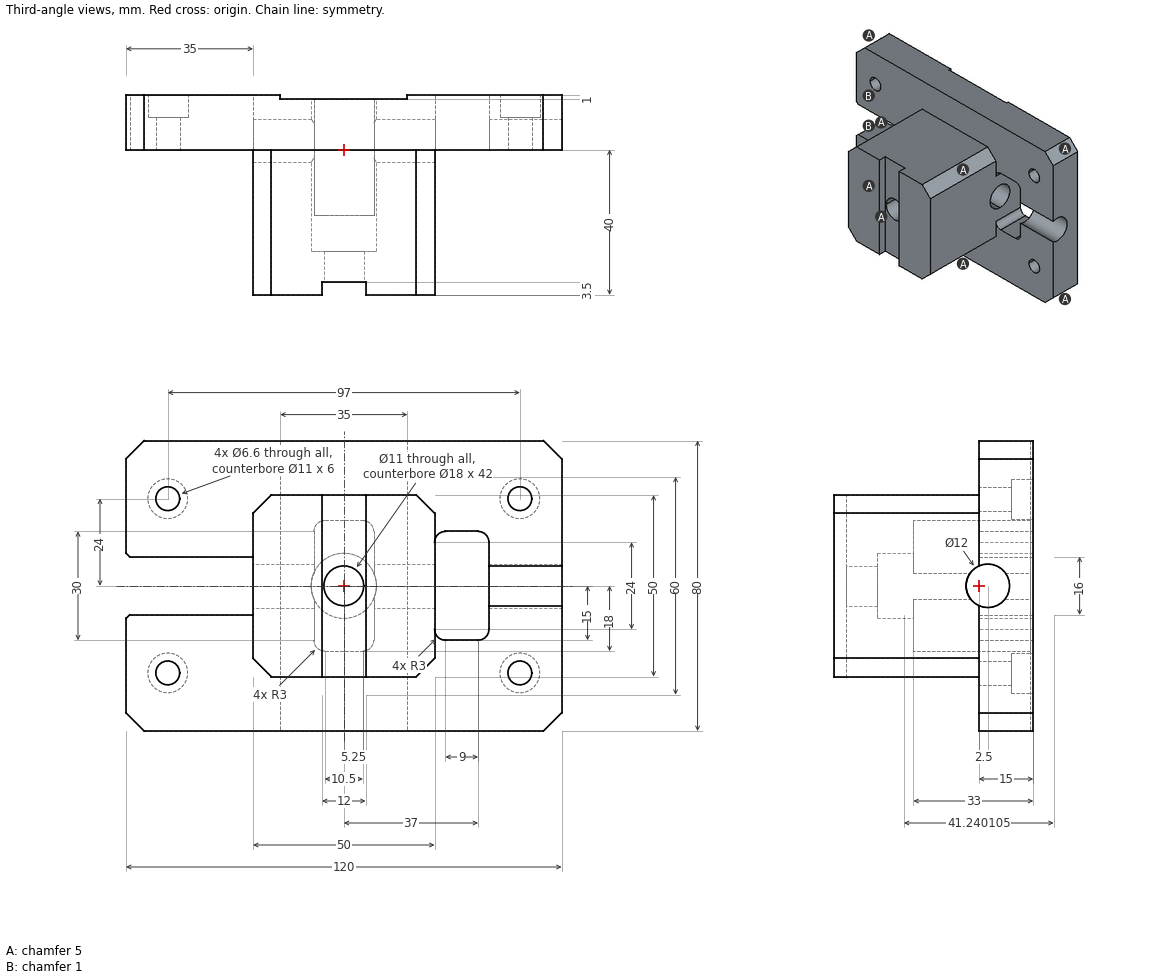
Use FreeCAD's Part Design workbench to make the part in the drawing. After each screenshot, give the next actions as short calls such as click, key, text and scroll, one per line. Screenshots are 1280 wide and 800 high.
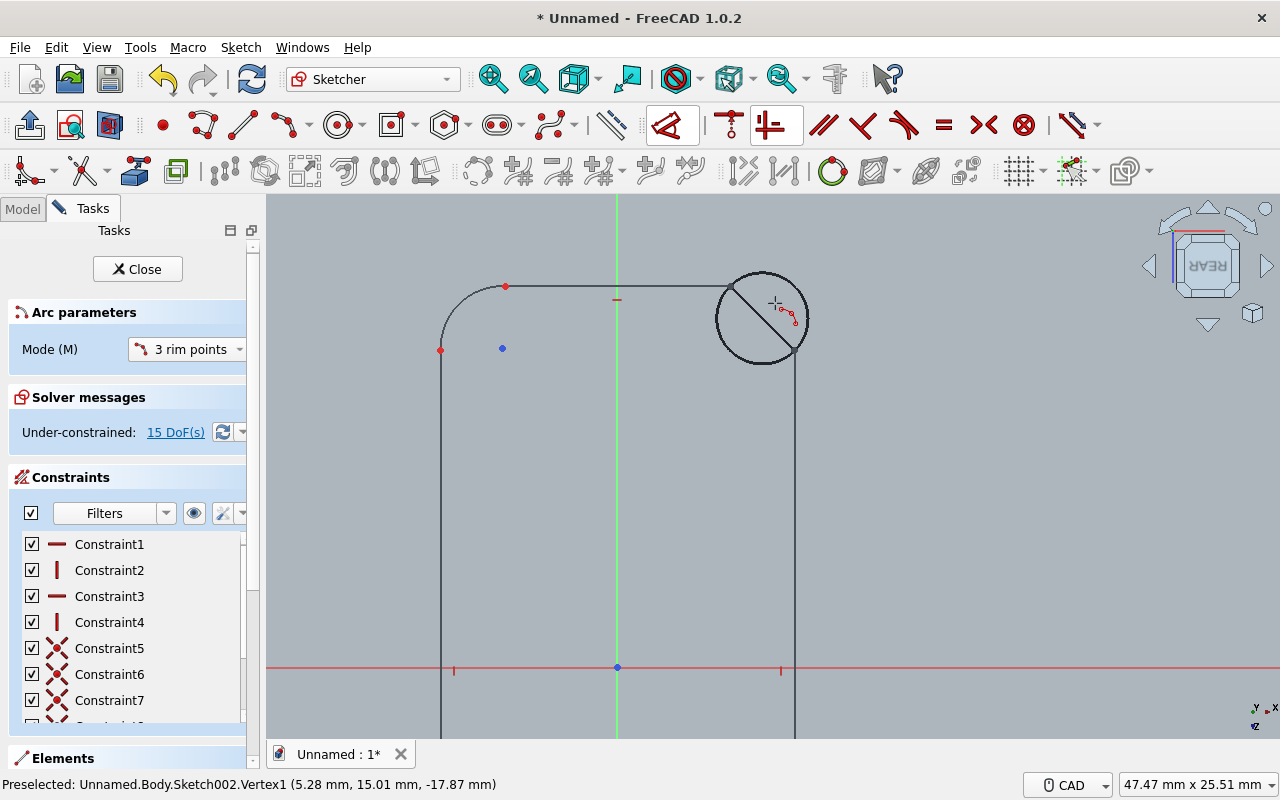
click(775, 302)
key(Escape)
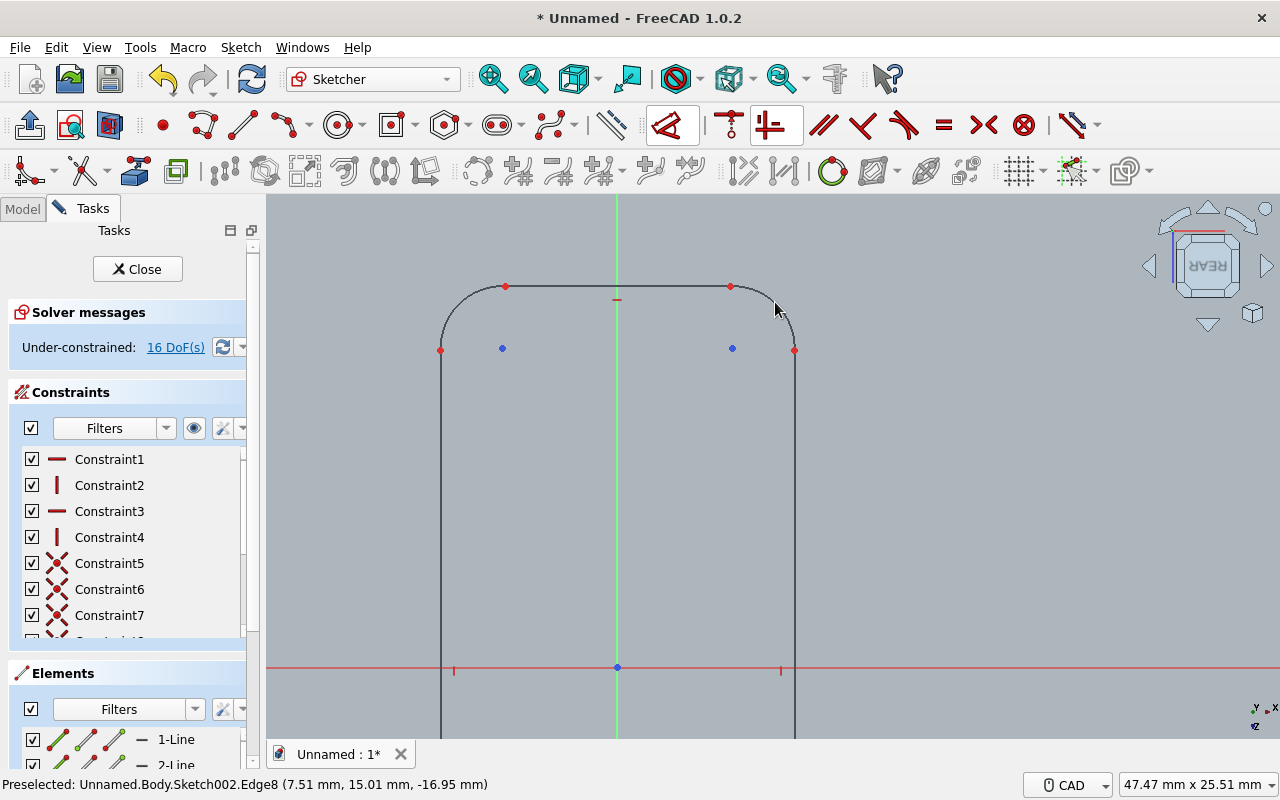
click(663, 286)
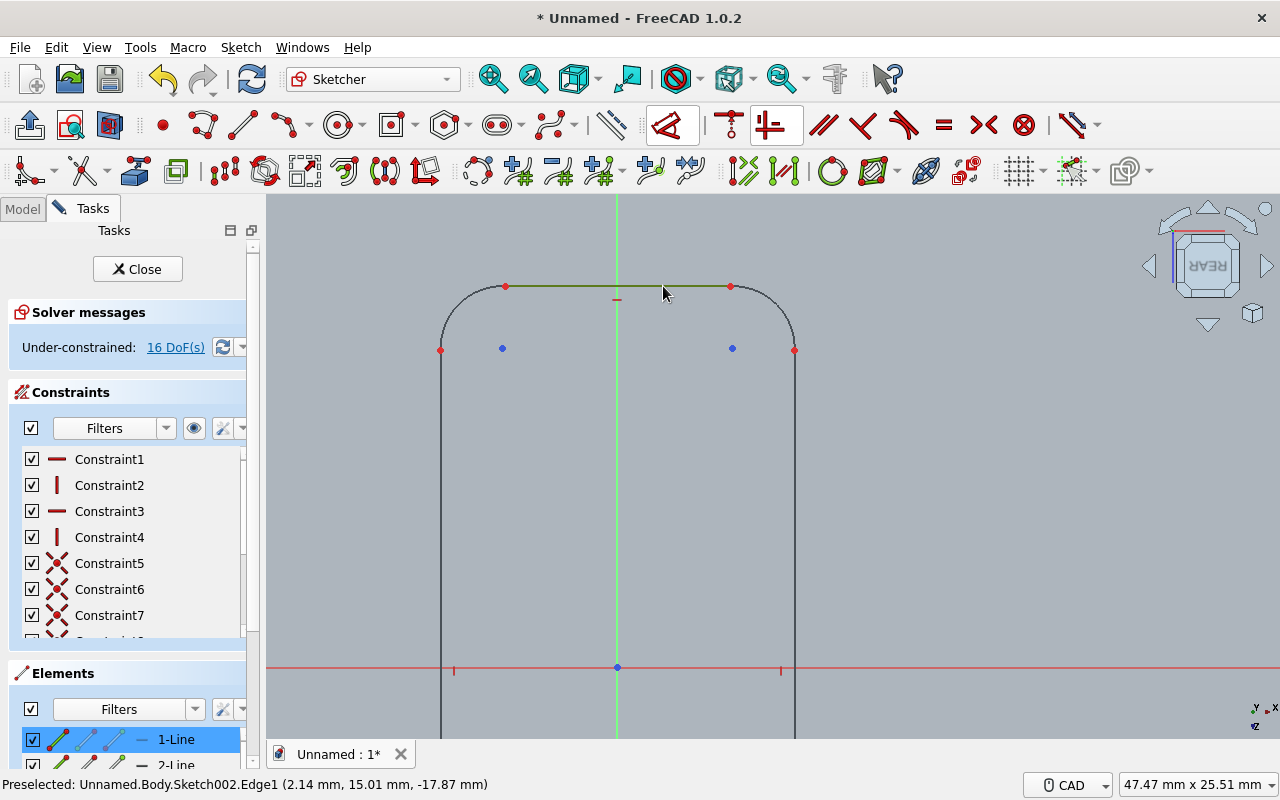
click(476, 292)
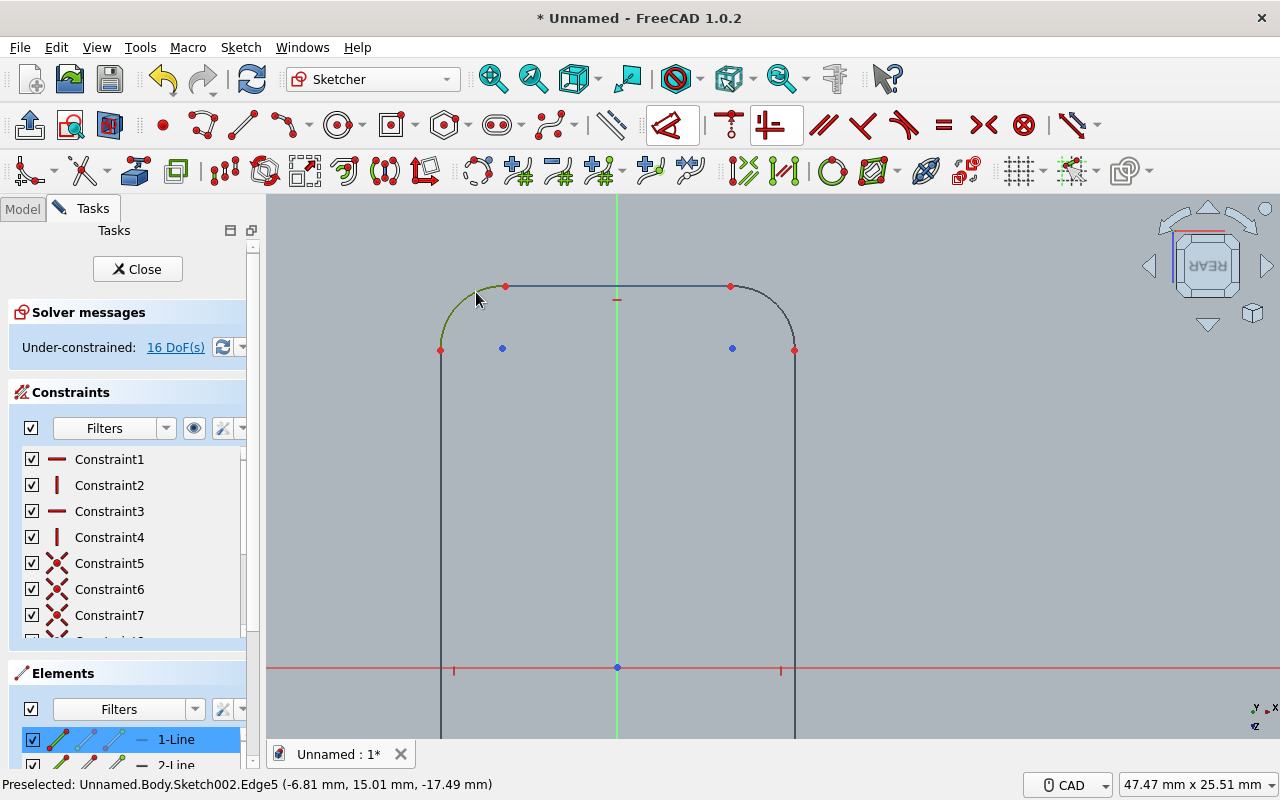
click(904, 126)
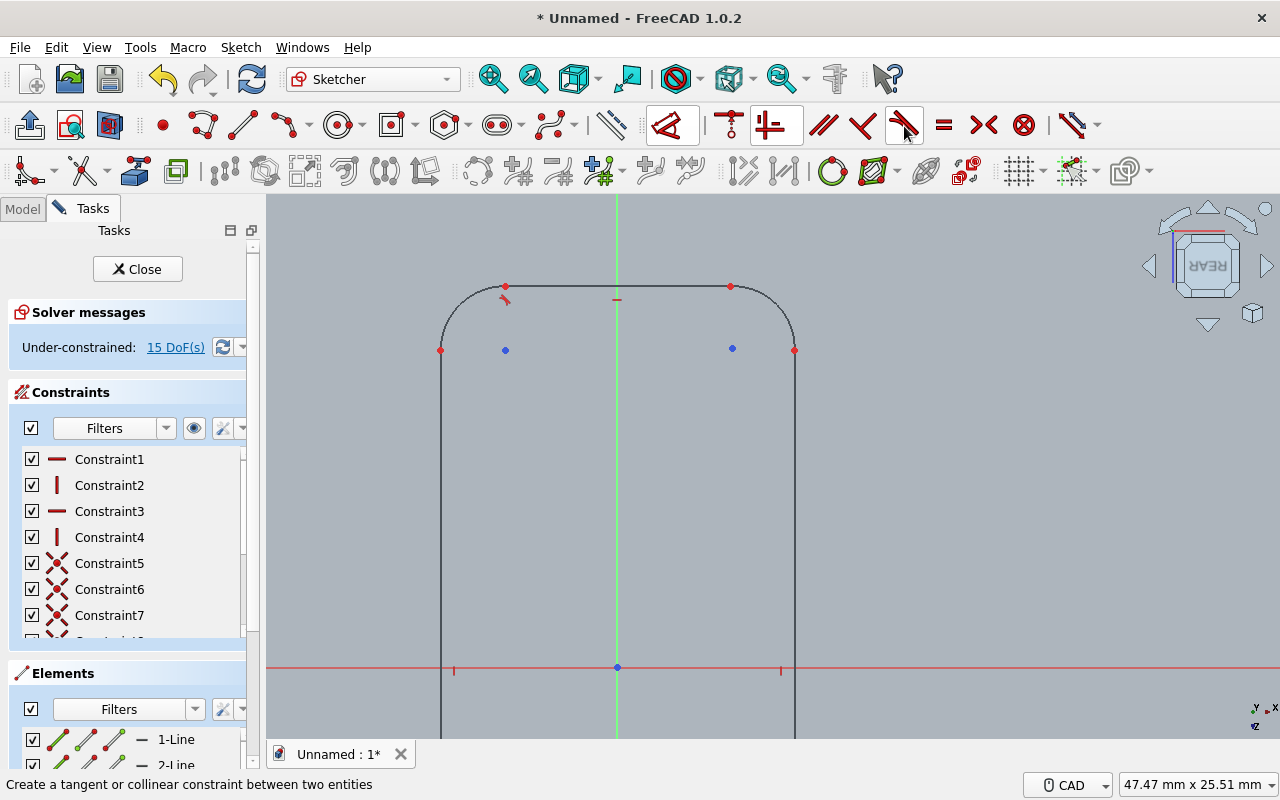
click(663, 286)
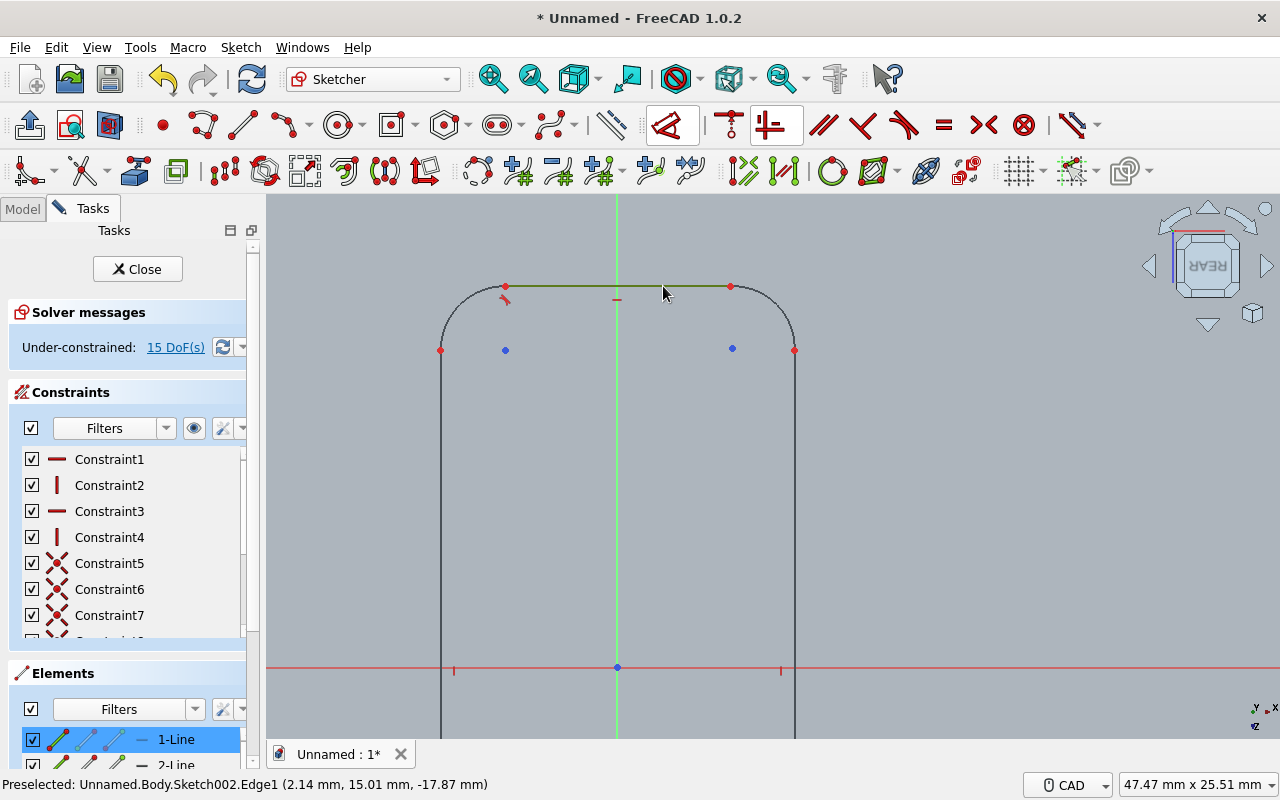
click(788, 321)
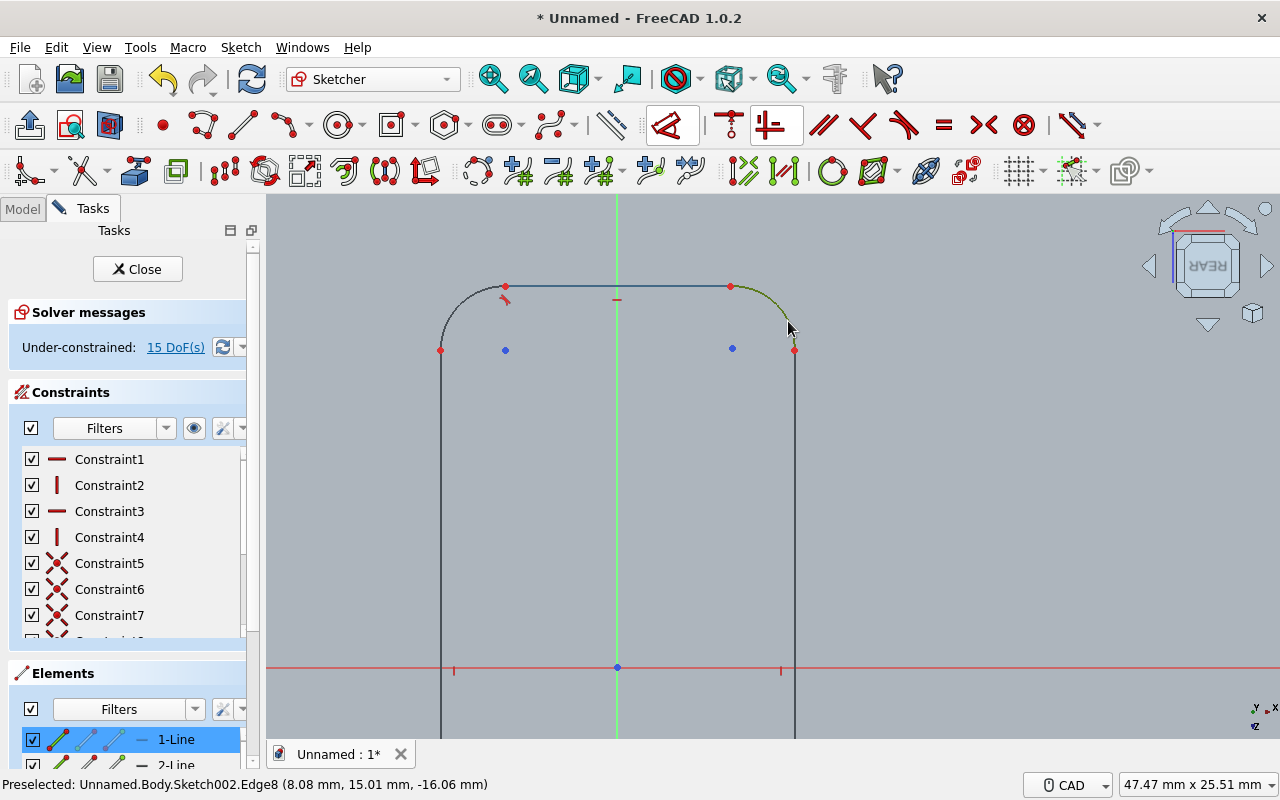
key(t)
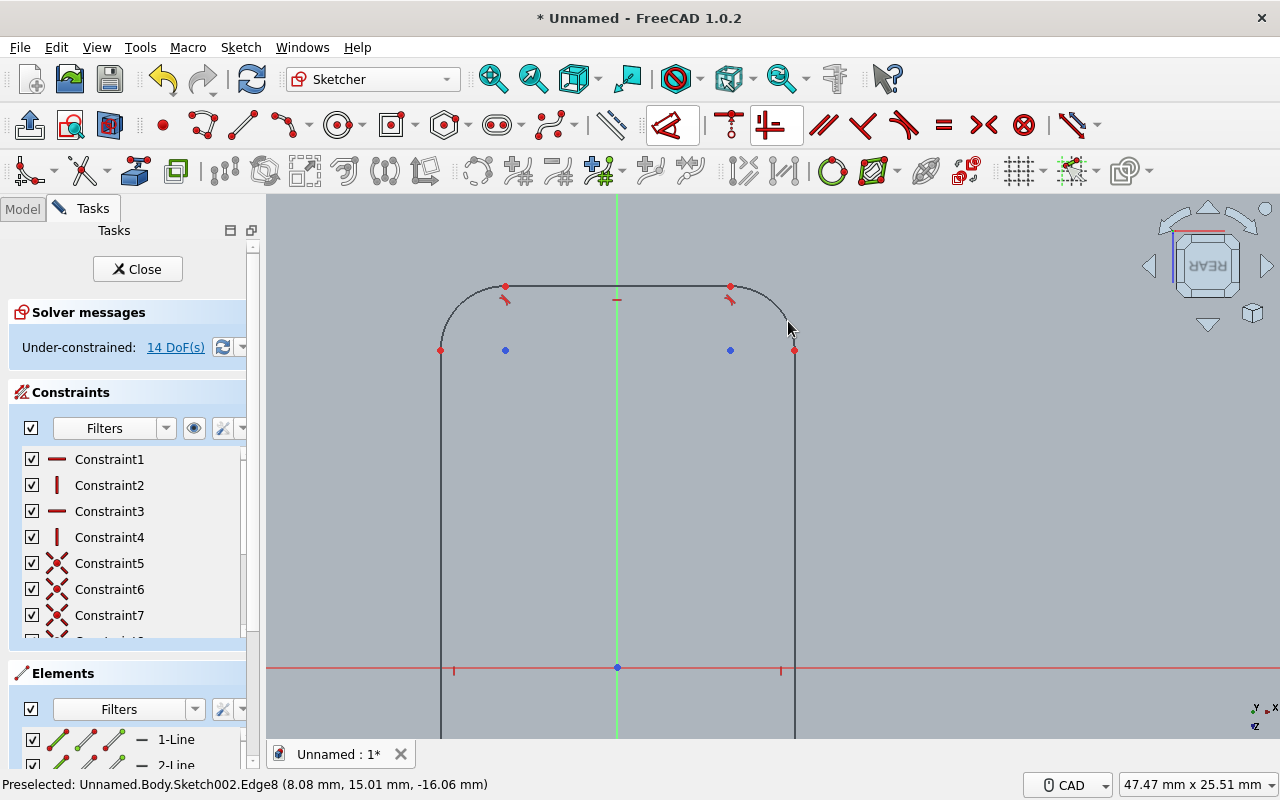
click(441, 542)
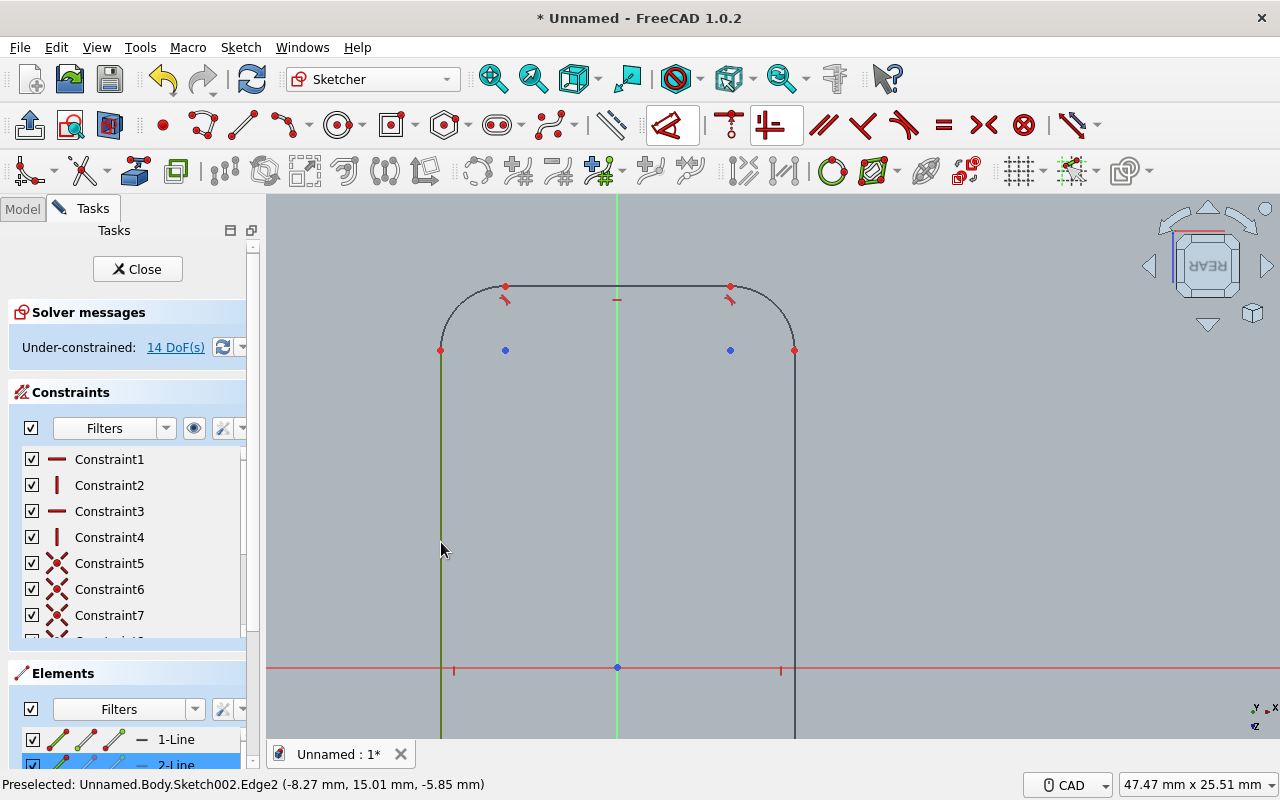
click(476, 293)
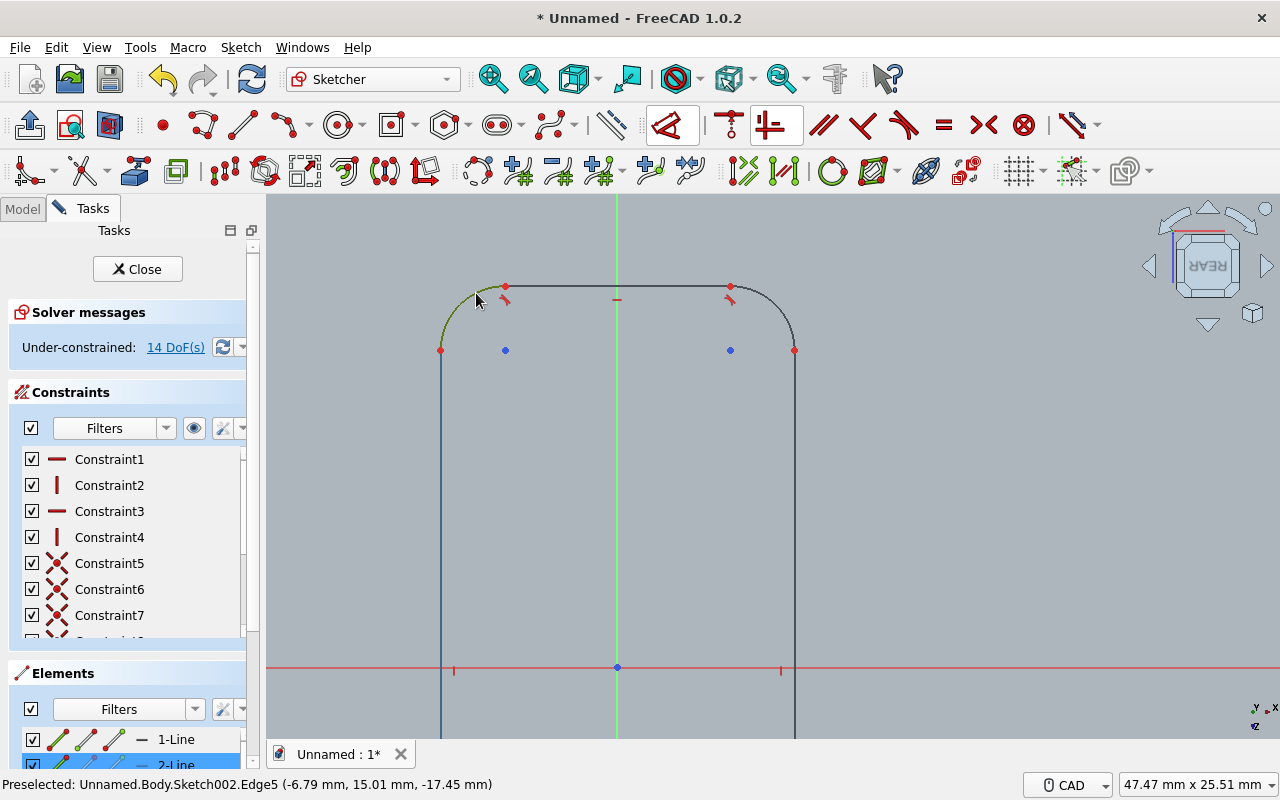
key(t)